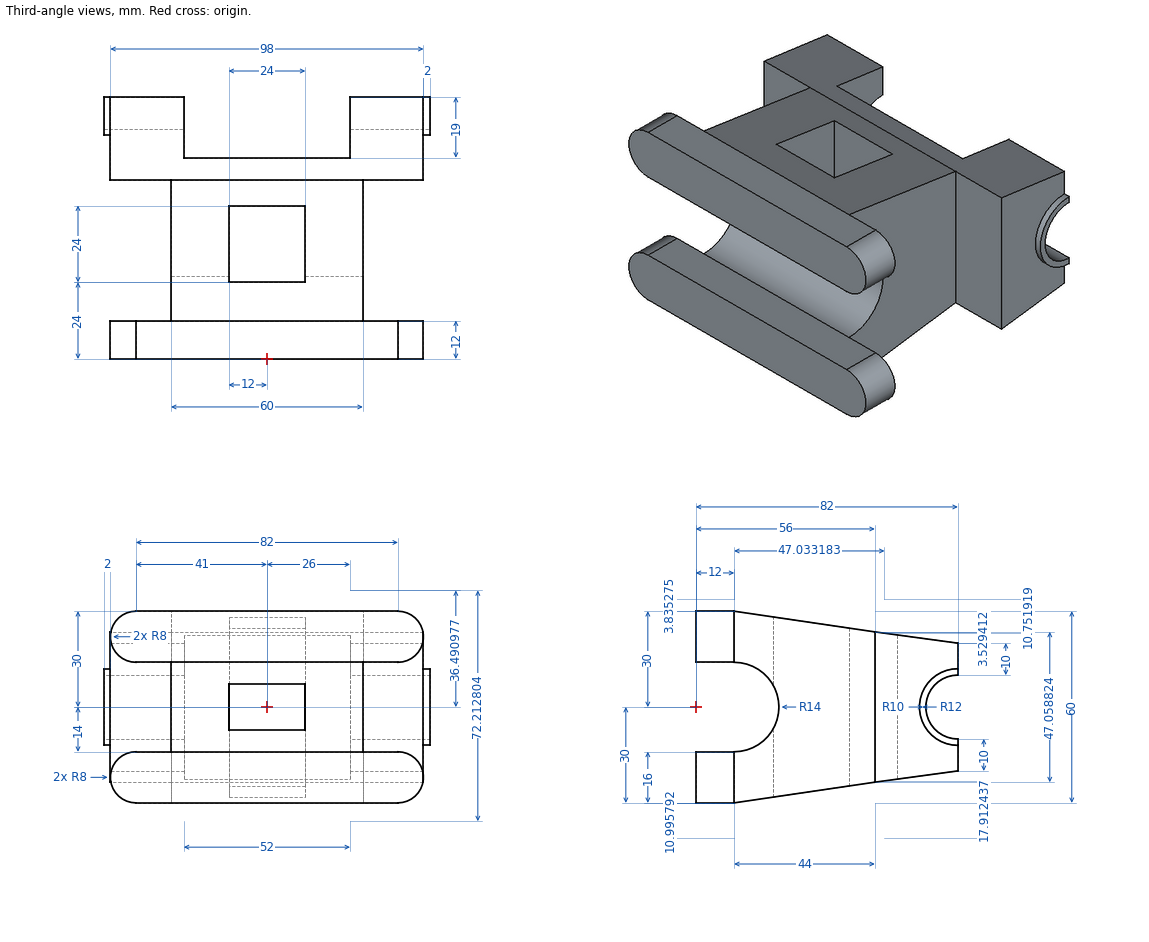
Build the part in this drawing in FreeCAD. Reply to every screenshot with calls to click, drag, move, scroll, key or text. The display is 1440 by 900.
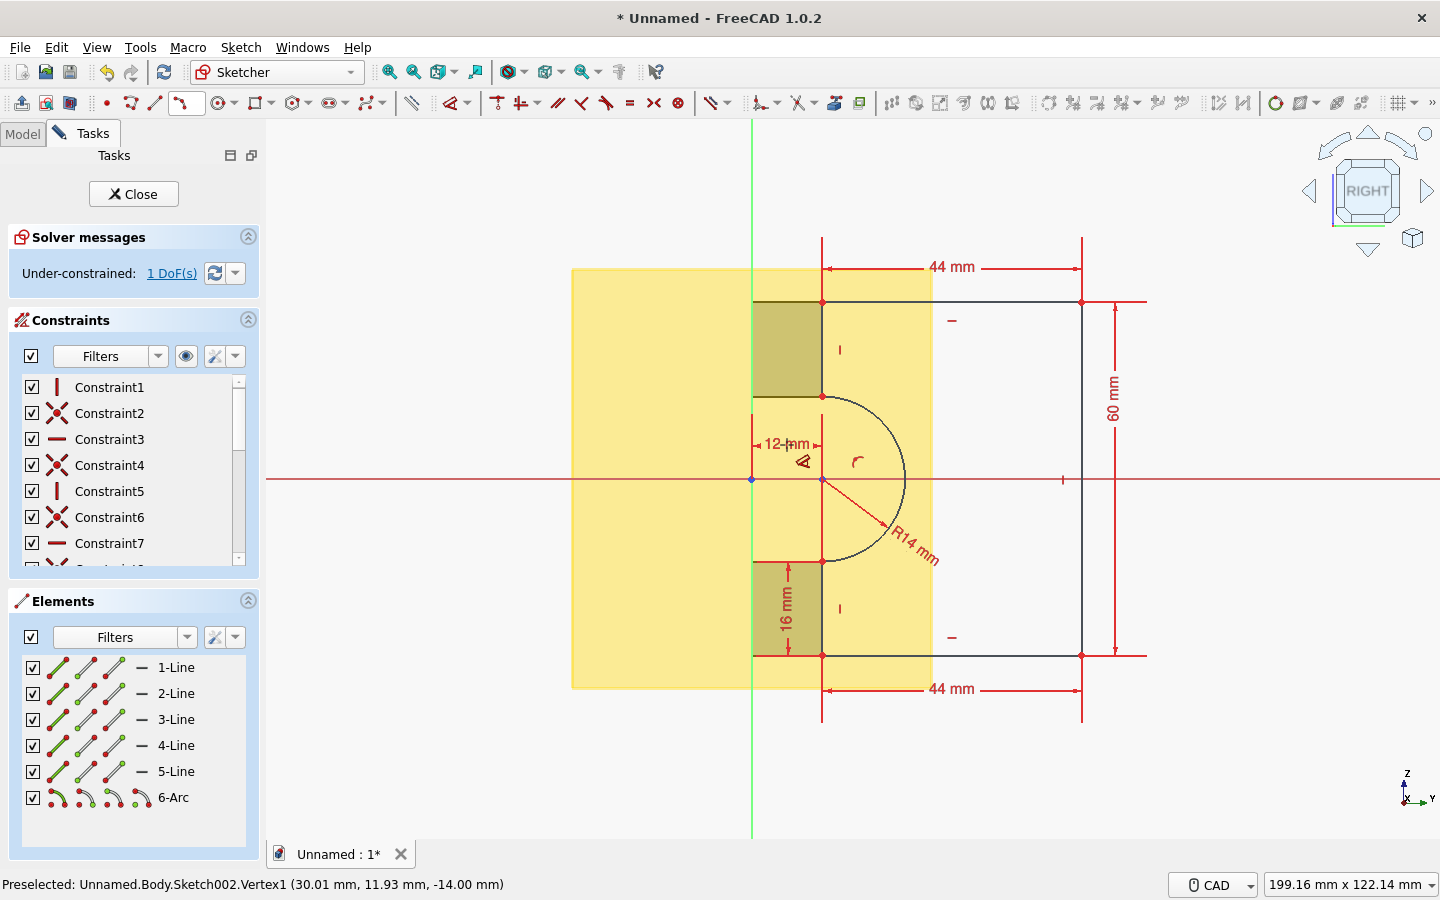
click(823, 479)
click(787, 513)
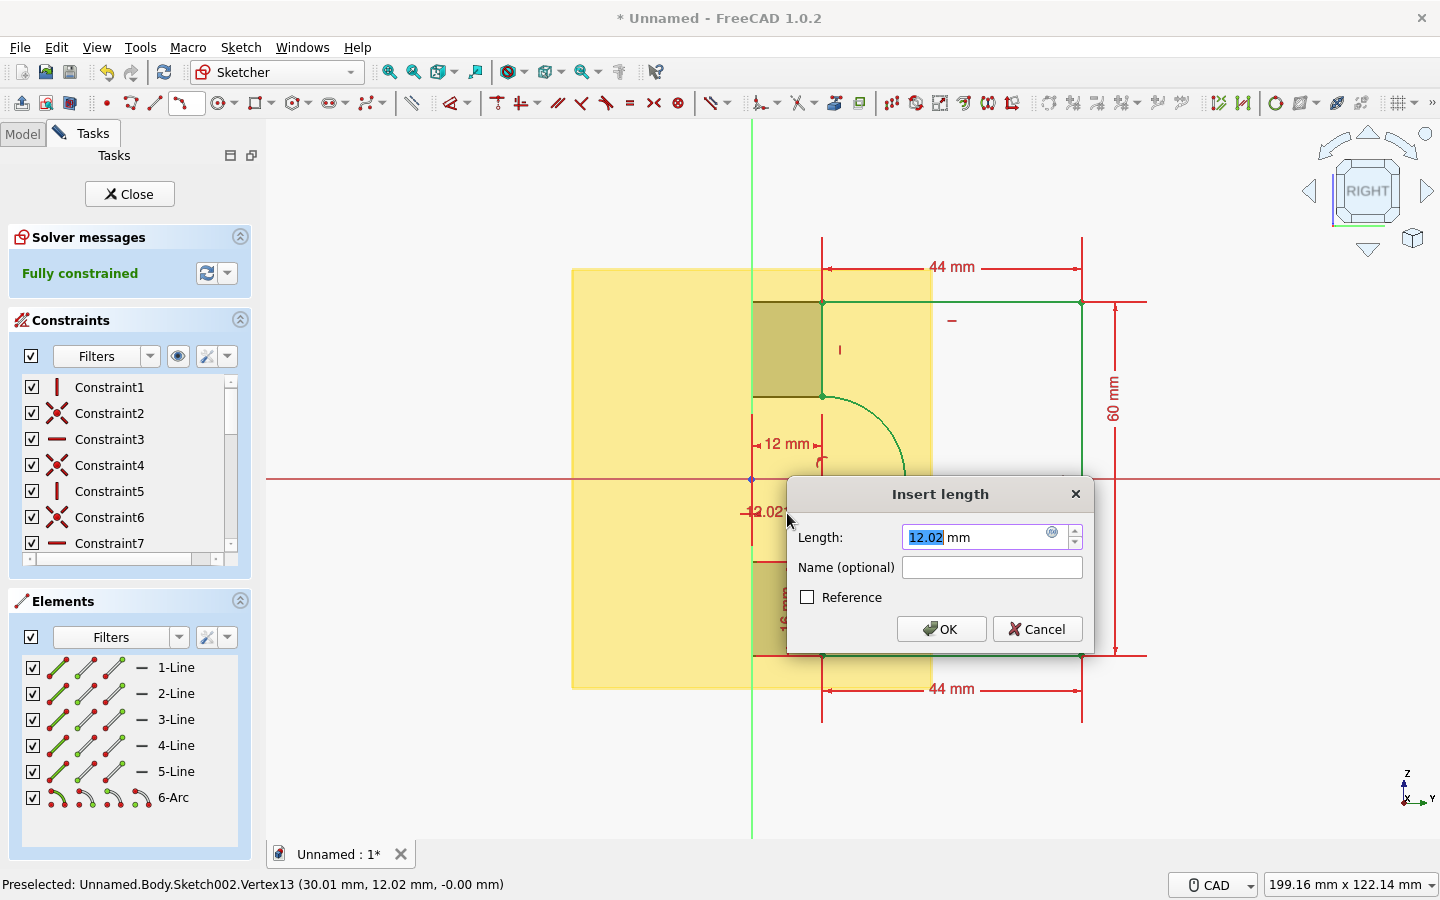
text(12)
key(Return)
key(Escape)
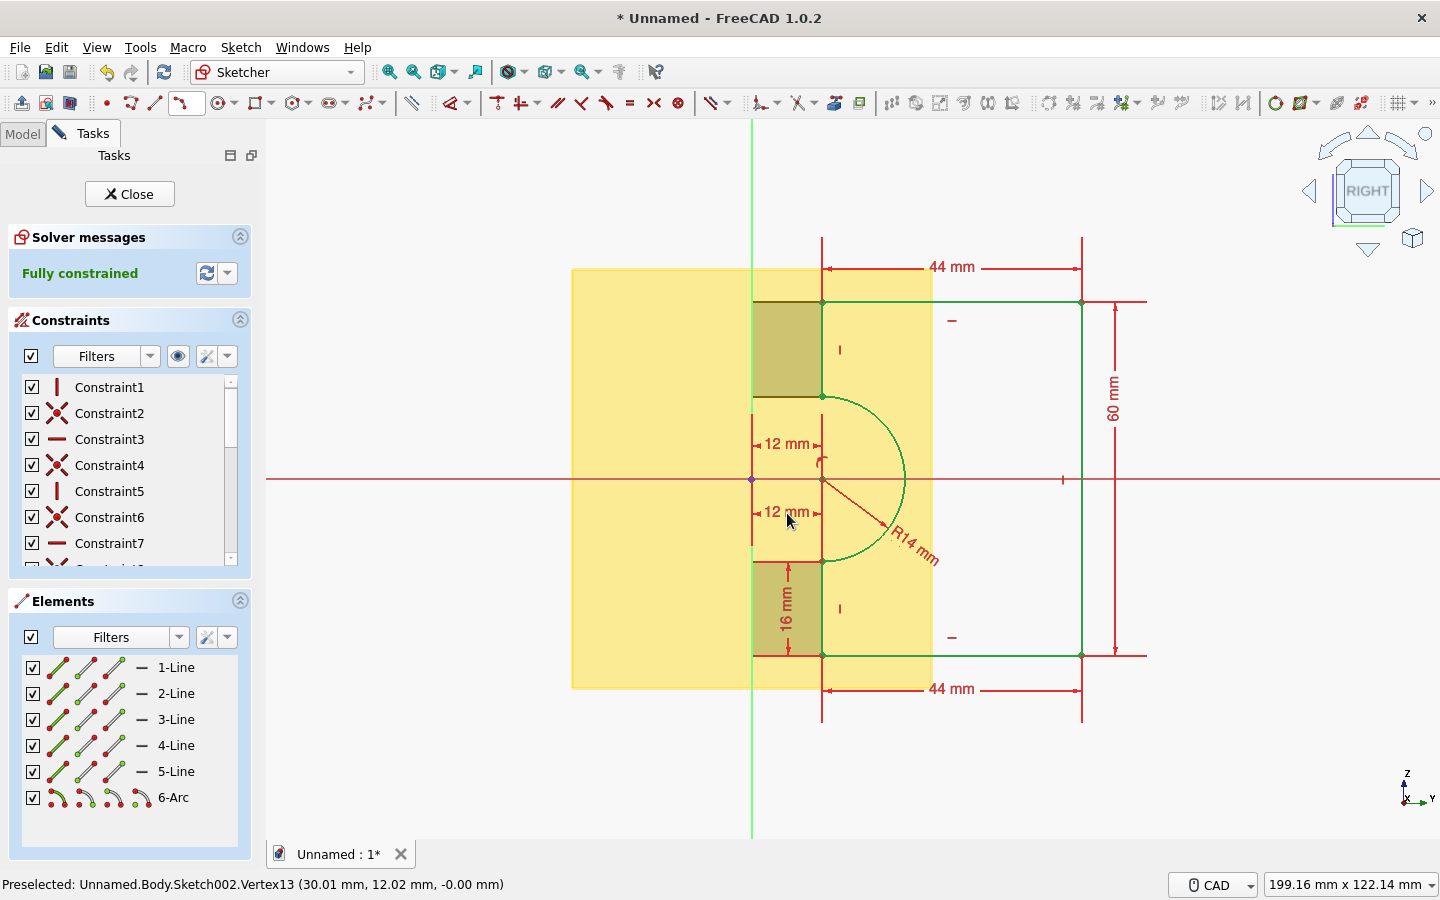
click(130, 194)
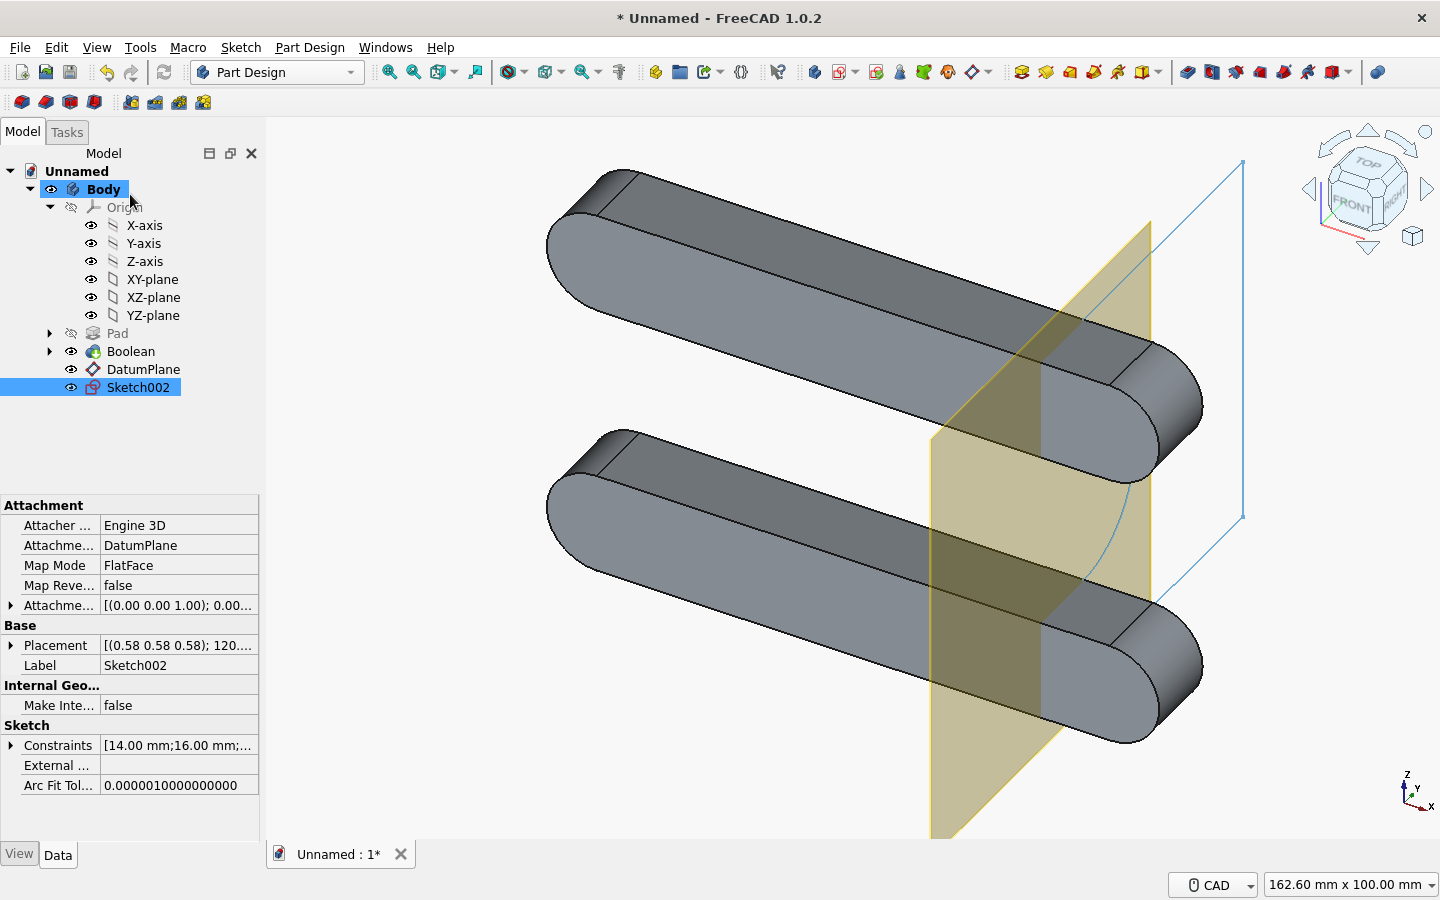
click(1022, 72)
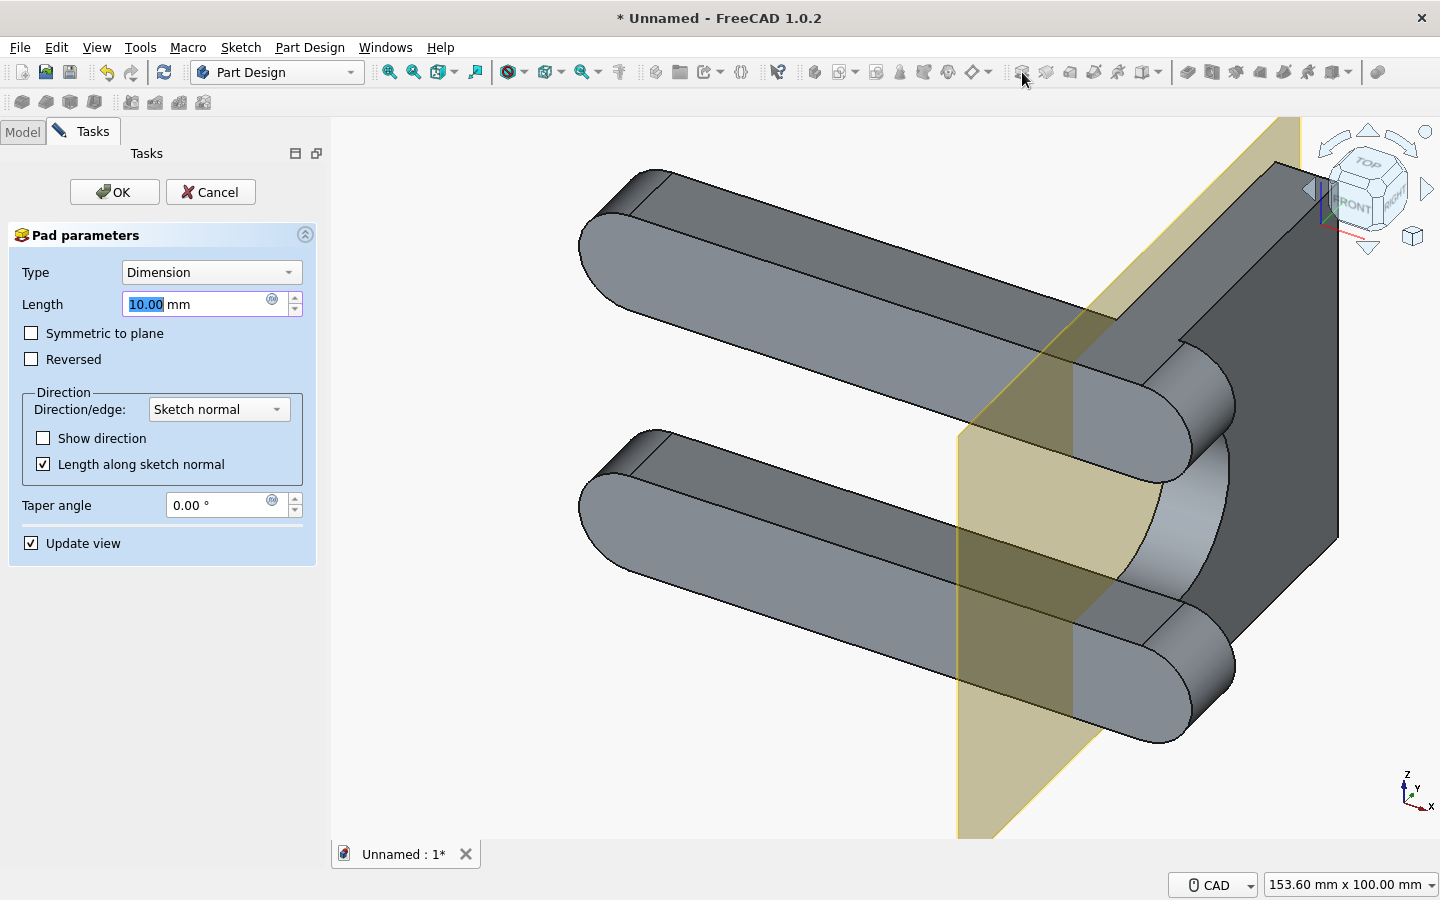
text(60)
key(Tab)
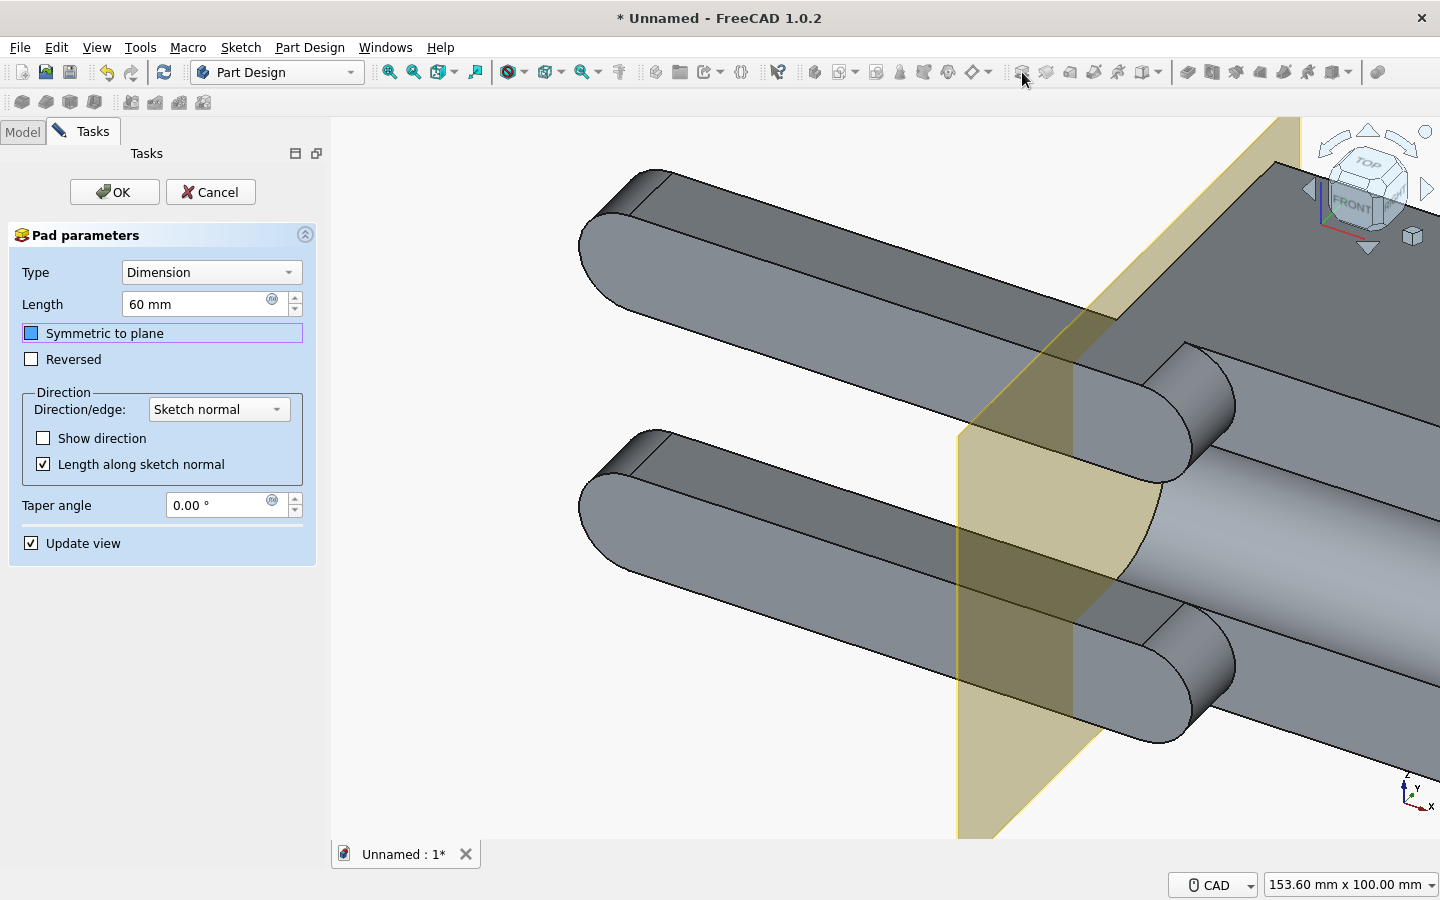
click(30, 359)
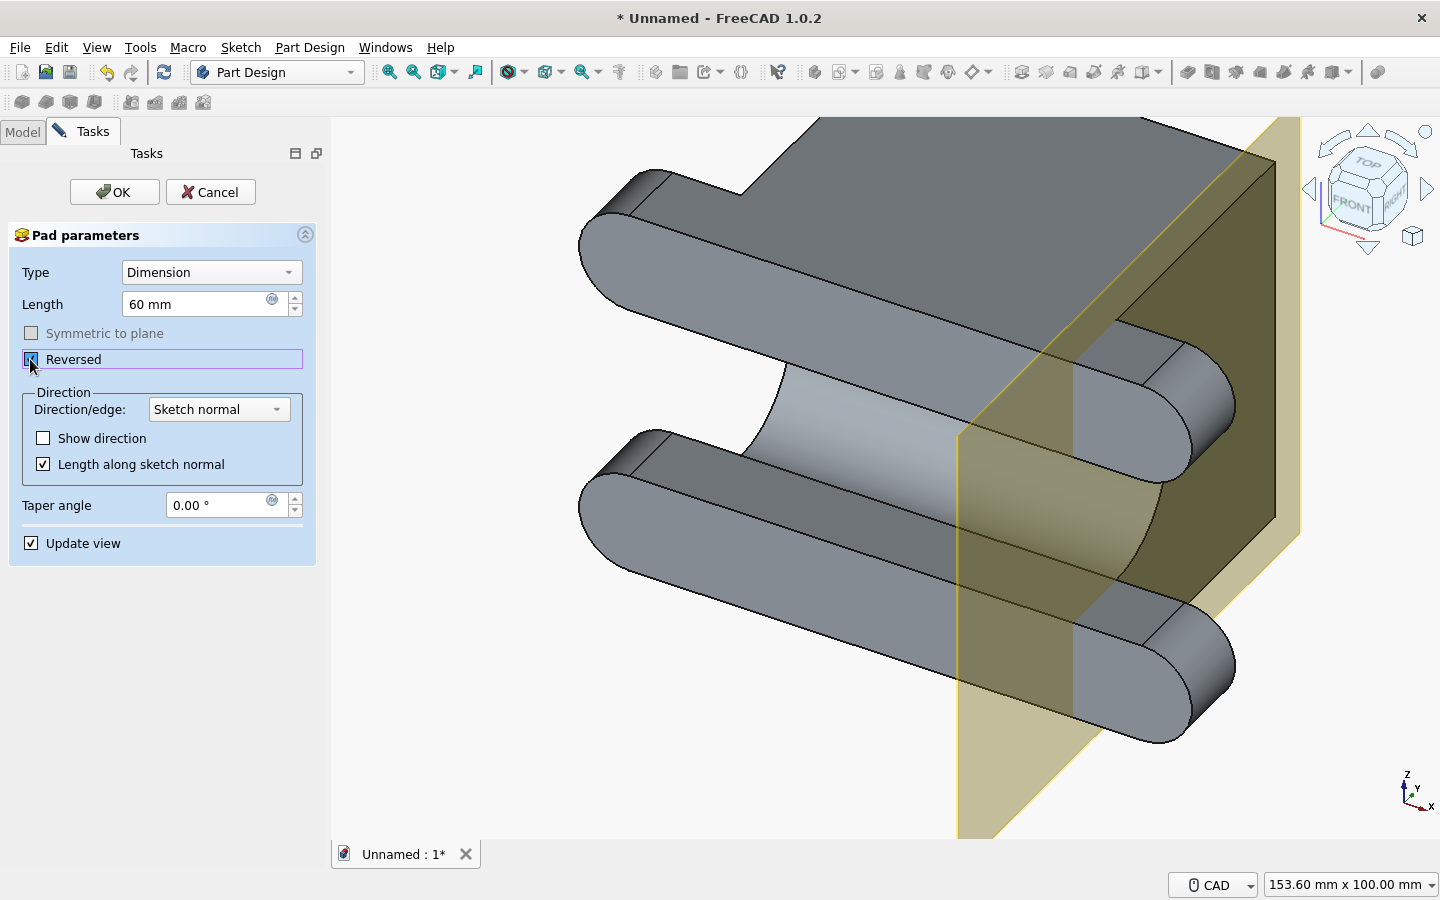
click(115, 192)